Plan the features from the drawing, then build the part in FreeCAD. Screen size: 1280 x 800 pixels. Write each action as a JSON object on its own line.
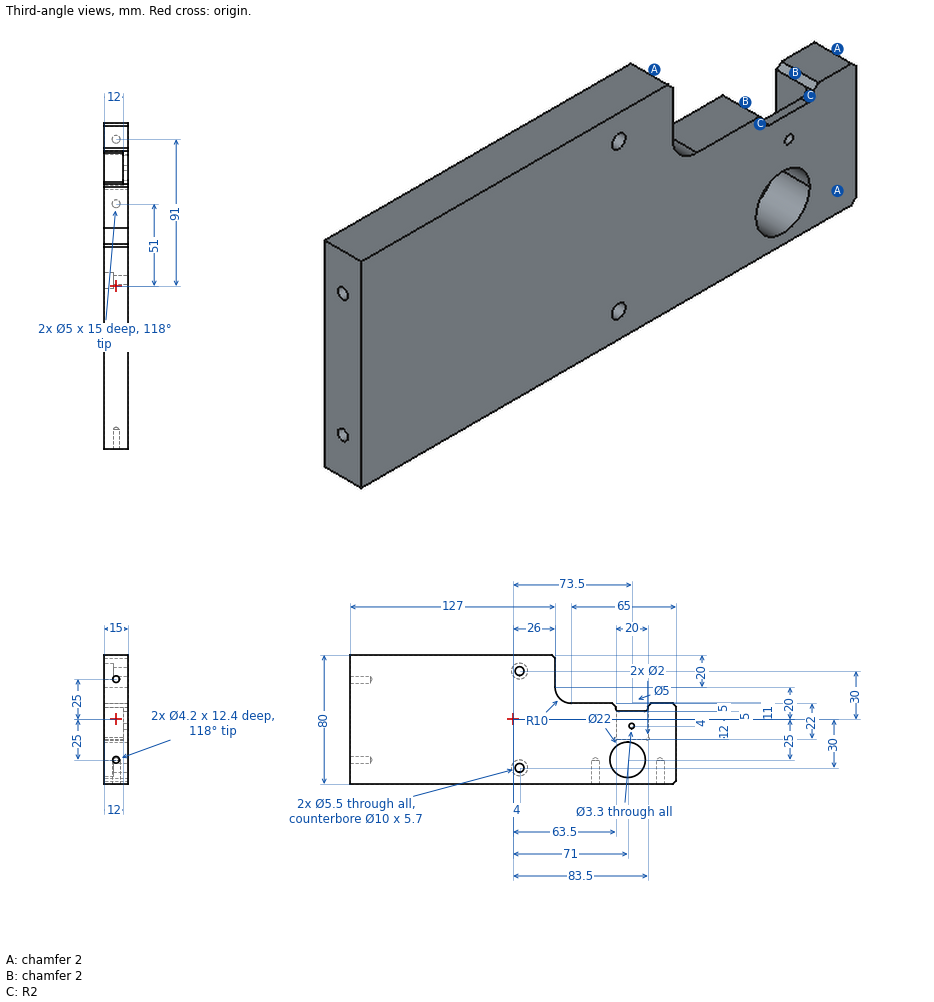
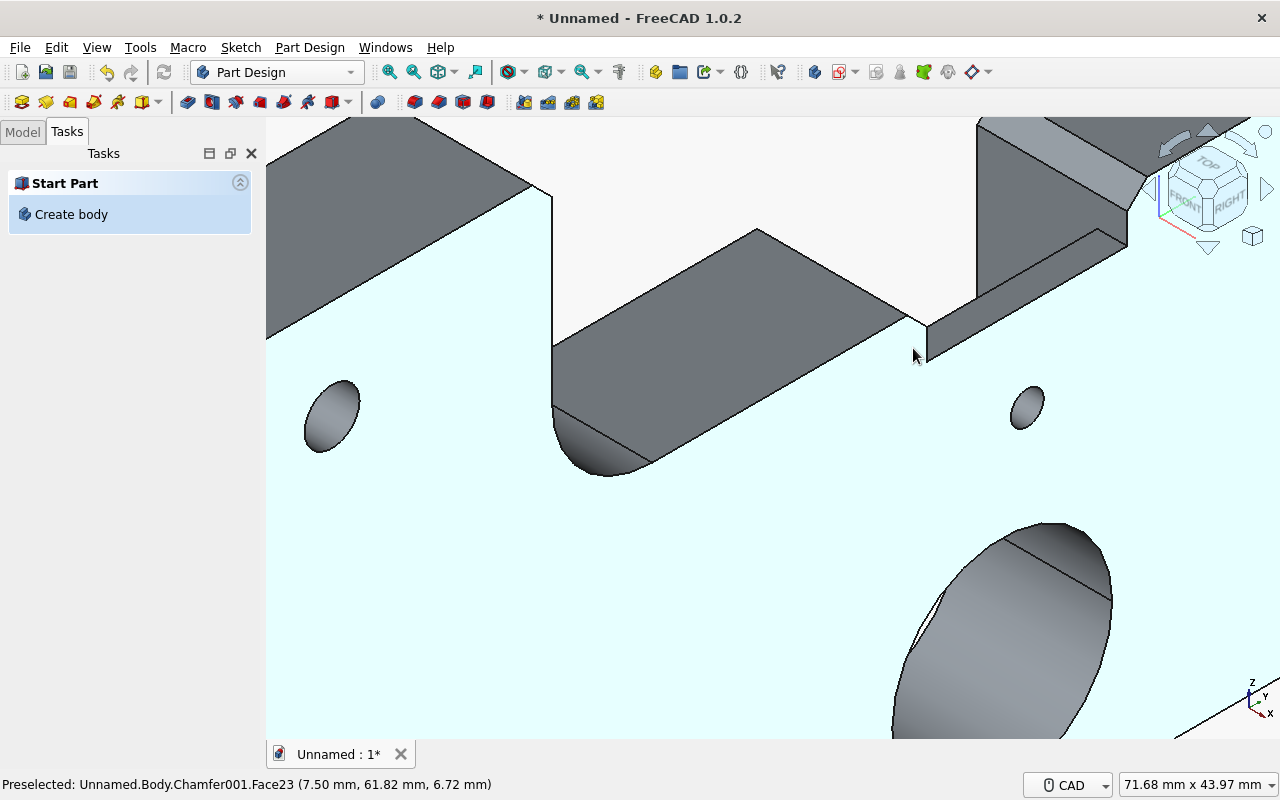
{"action": "left_click", "coordinate": [390, 72]}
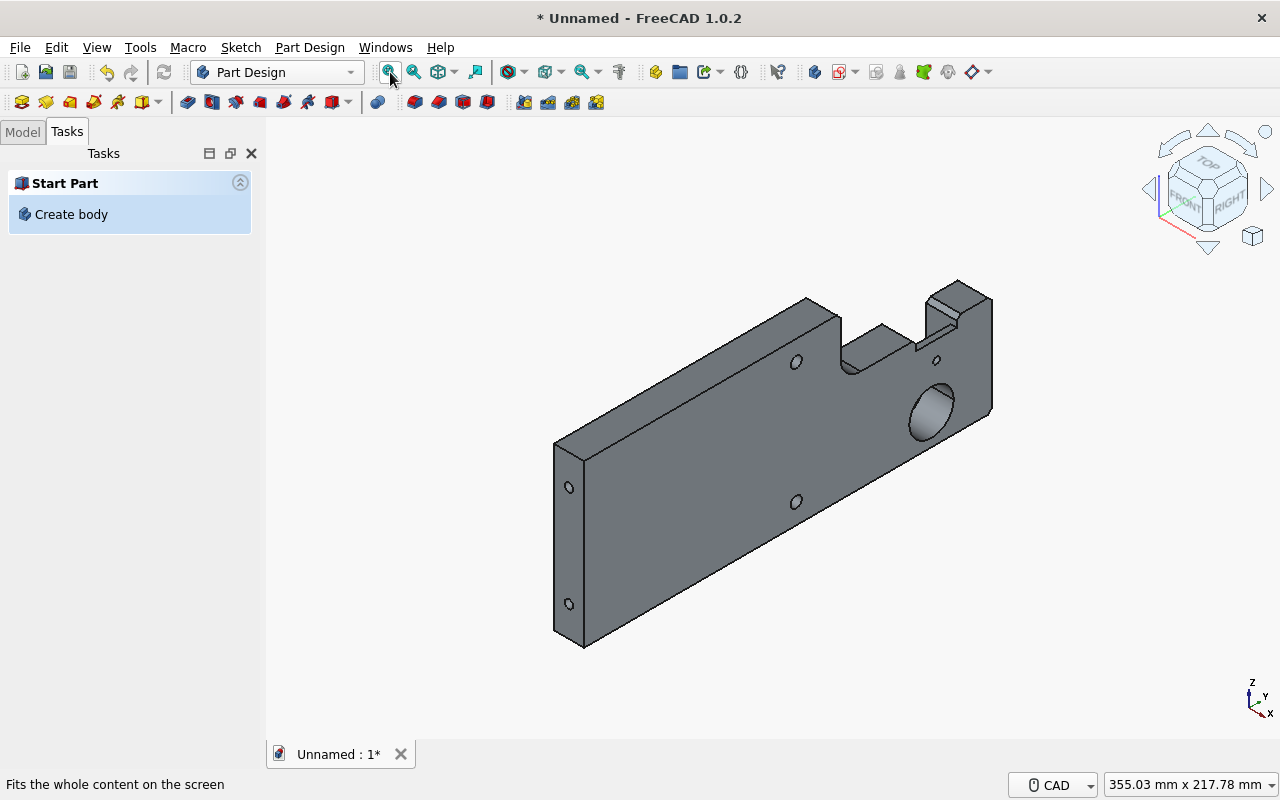
{"action": "key", "text": "2"}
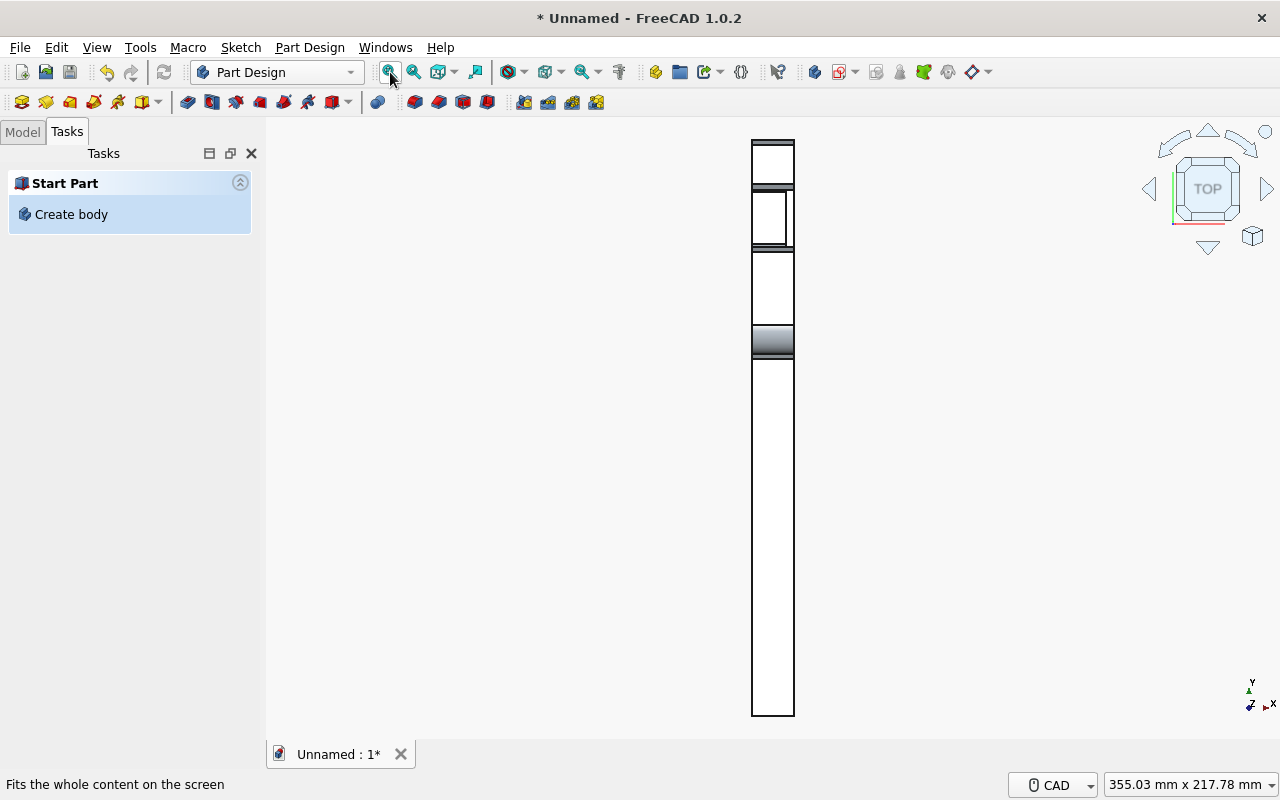
{"action": "scroll", "coordinate": [790, 246], "scroll_direction": "up", "scroll_amount": 8}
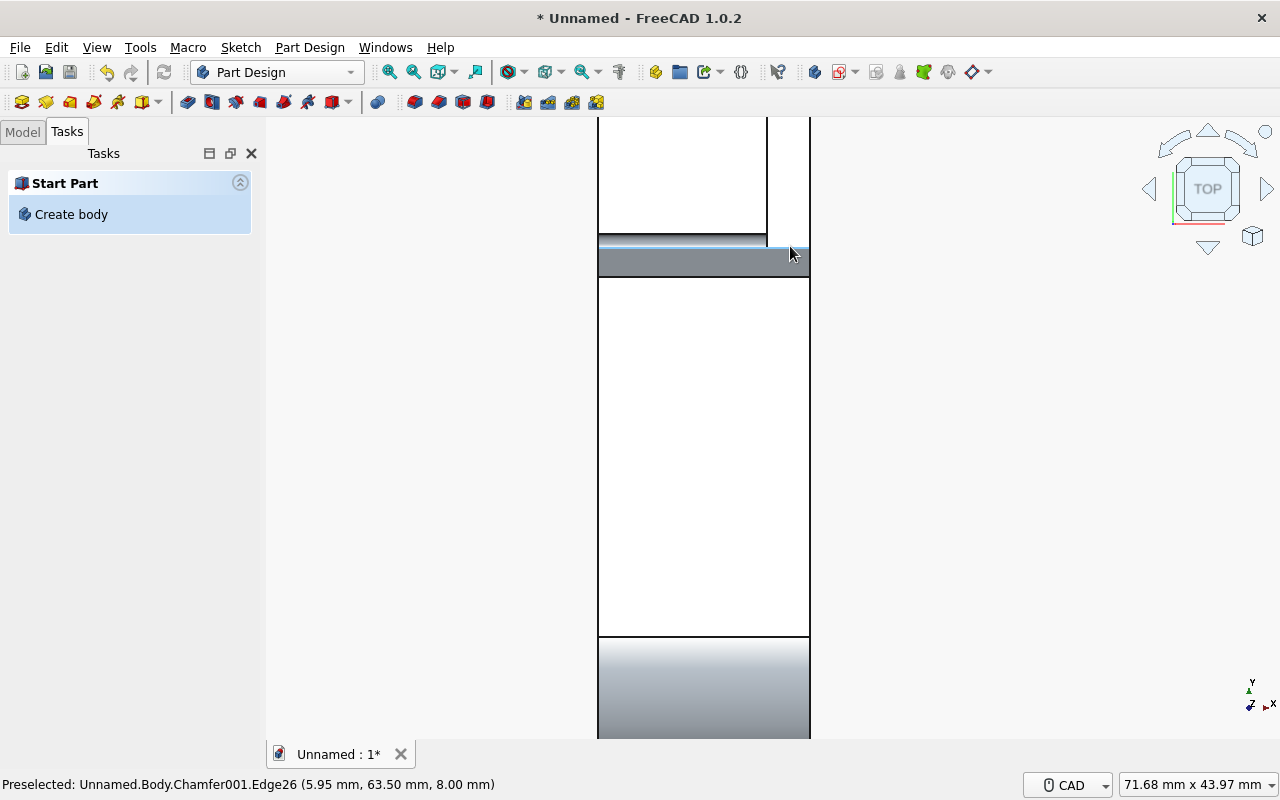
{"action": "left_click", "coordinate": [390, 72]}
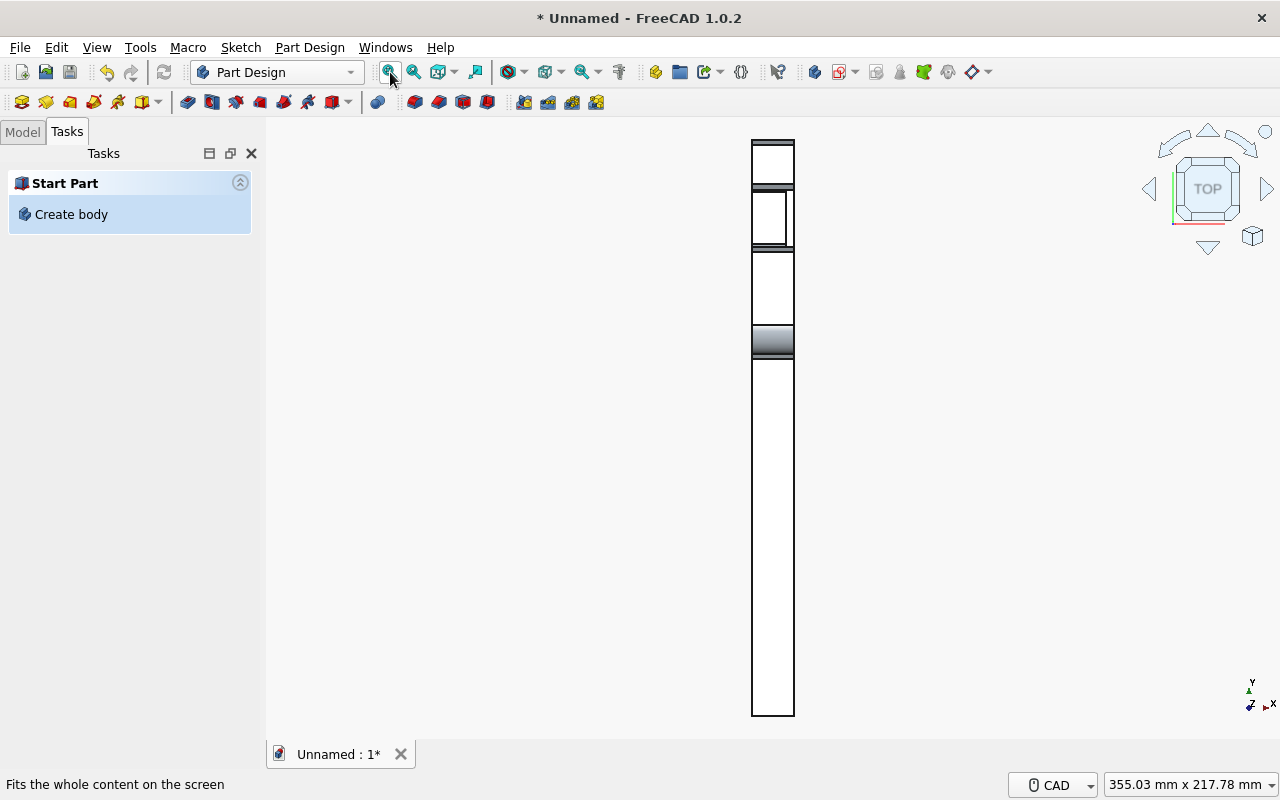
{"action": "key", "text": "1"}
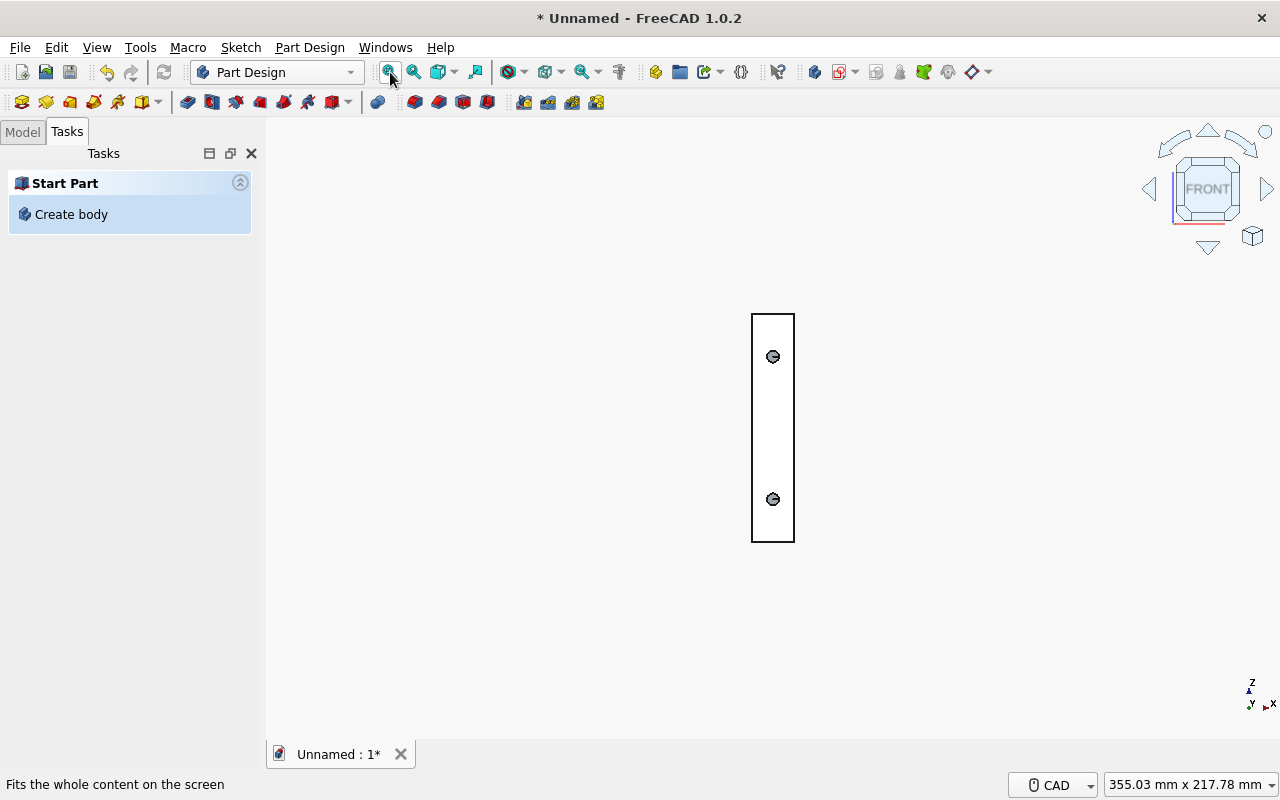
{"action": "left_click", "coordinate": [390, 72]}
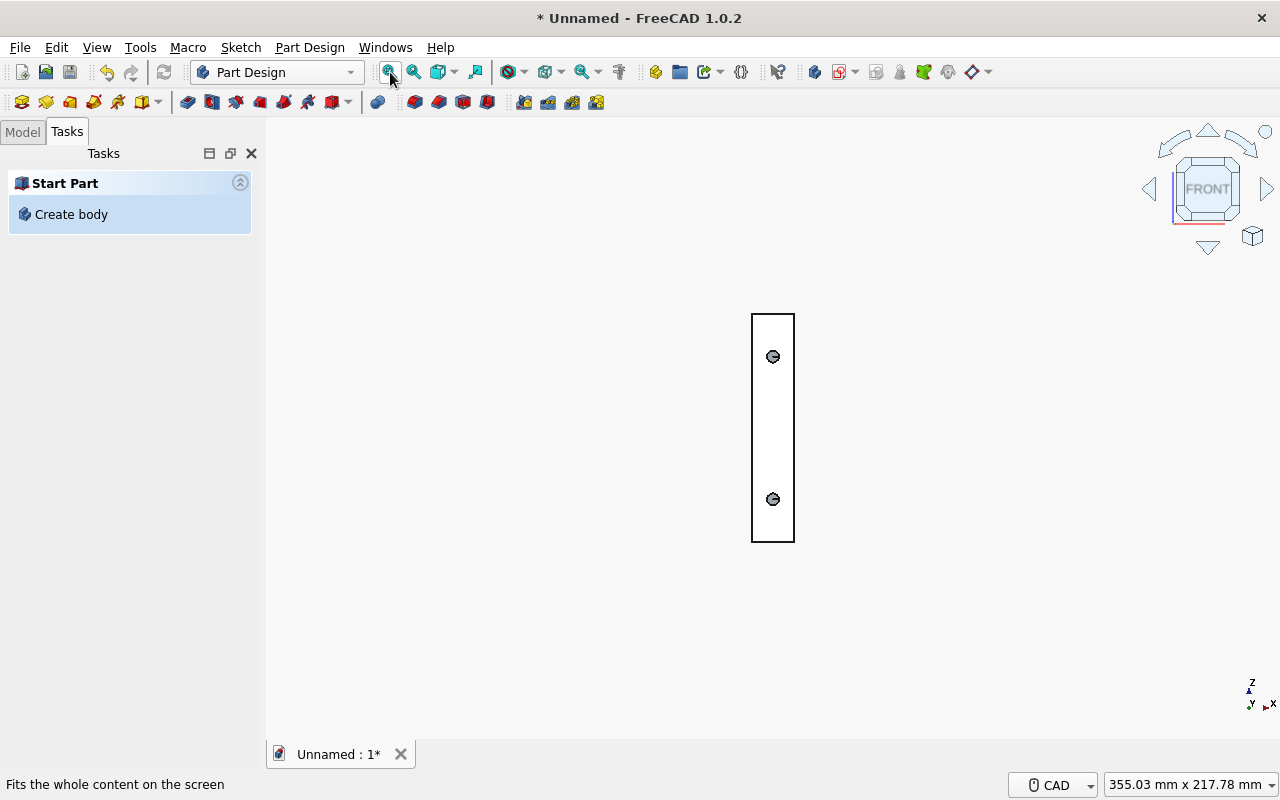
{"action": "scroll", "coordinate": [790, 413], "scroll_direction": "up", "scroll_amount": 8}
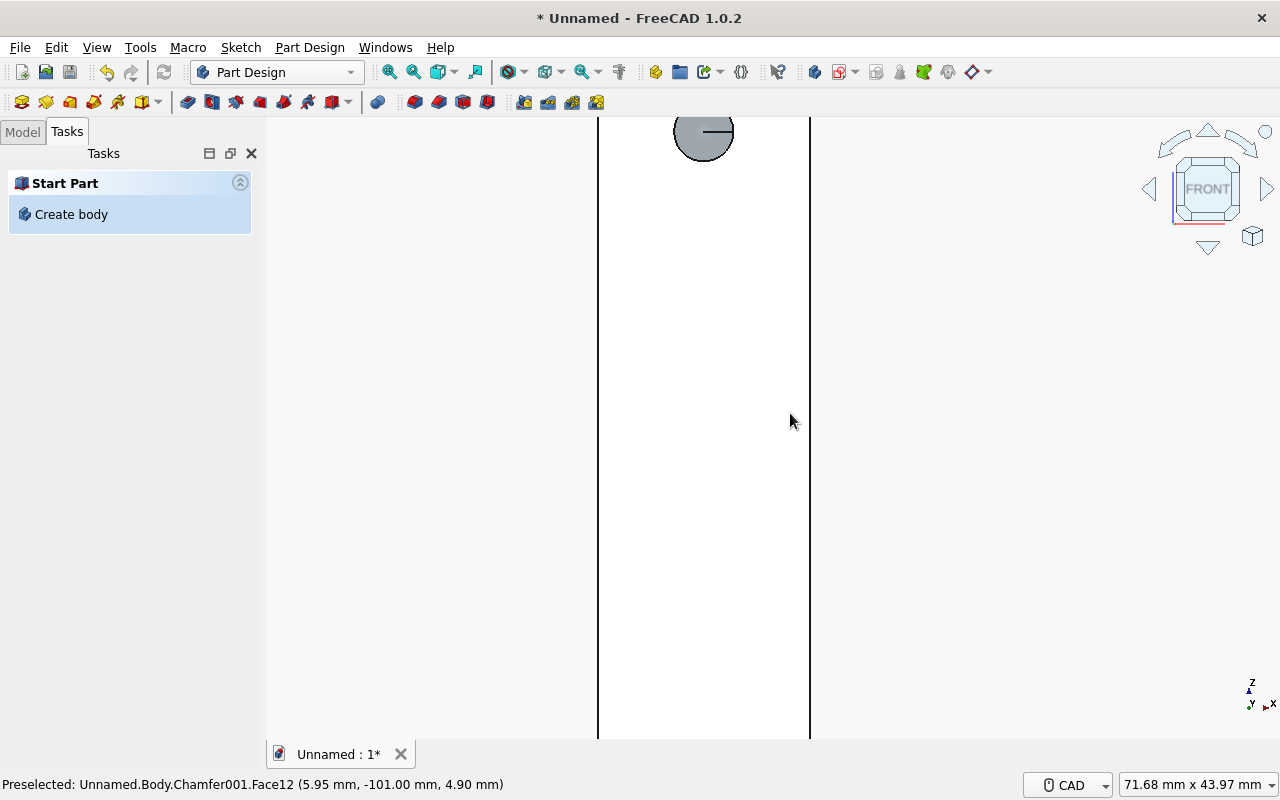
{"action": "left_click", "coordinate": [390, 72]}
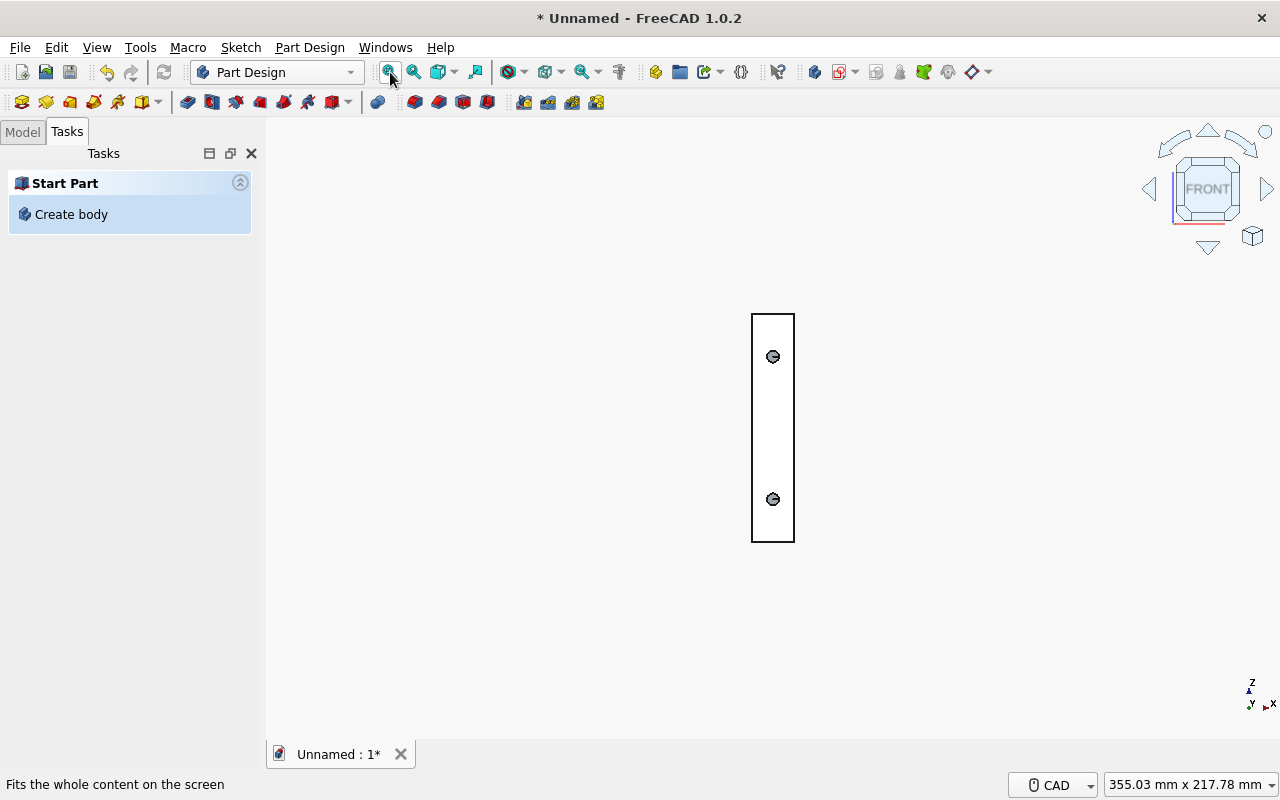
{"action": "key", "text": "3"}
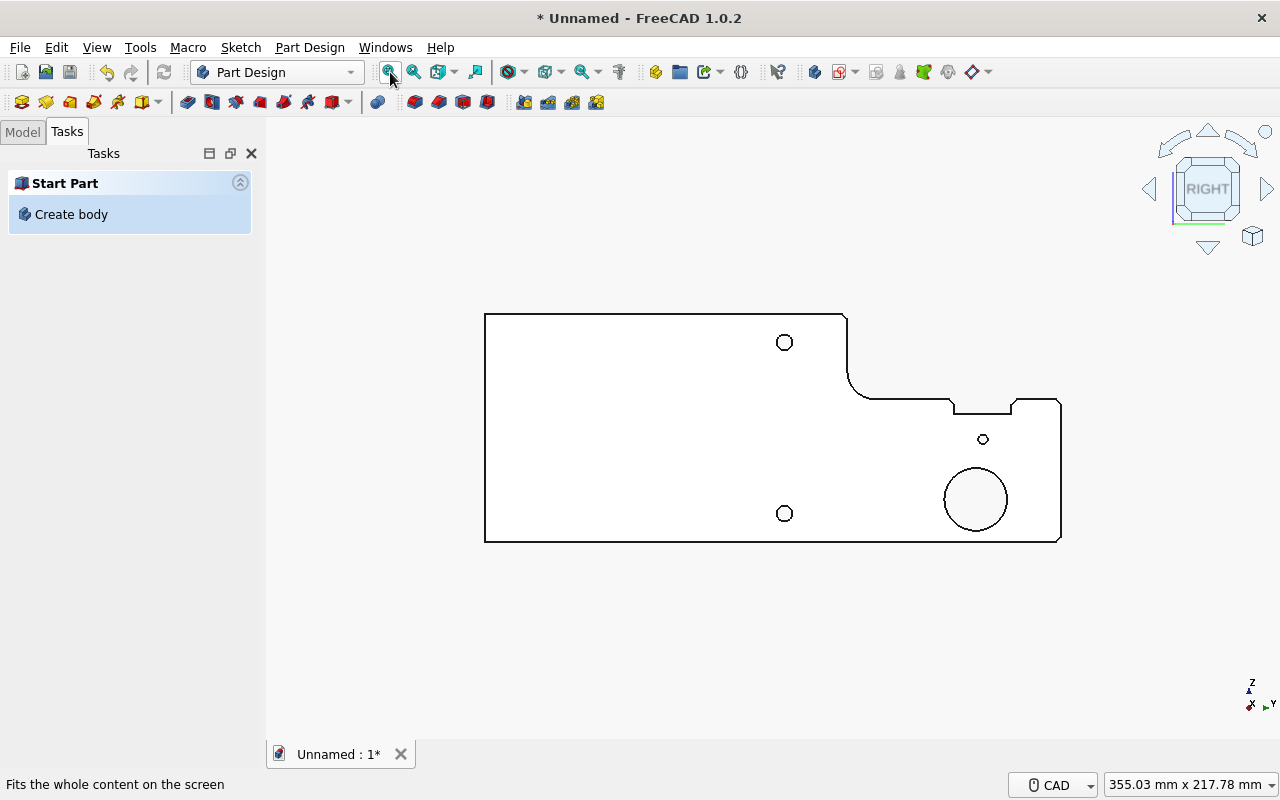
{"action": "scroll", "coordinate": [954, 413], "scroll_direction": "up", "scroll_amount": 8}